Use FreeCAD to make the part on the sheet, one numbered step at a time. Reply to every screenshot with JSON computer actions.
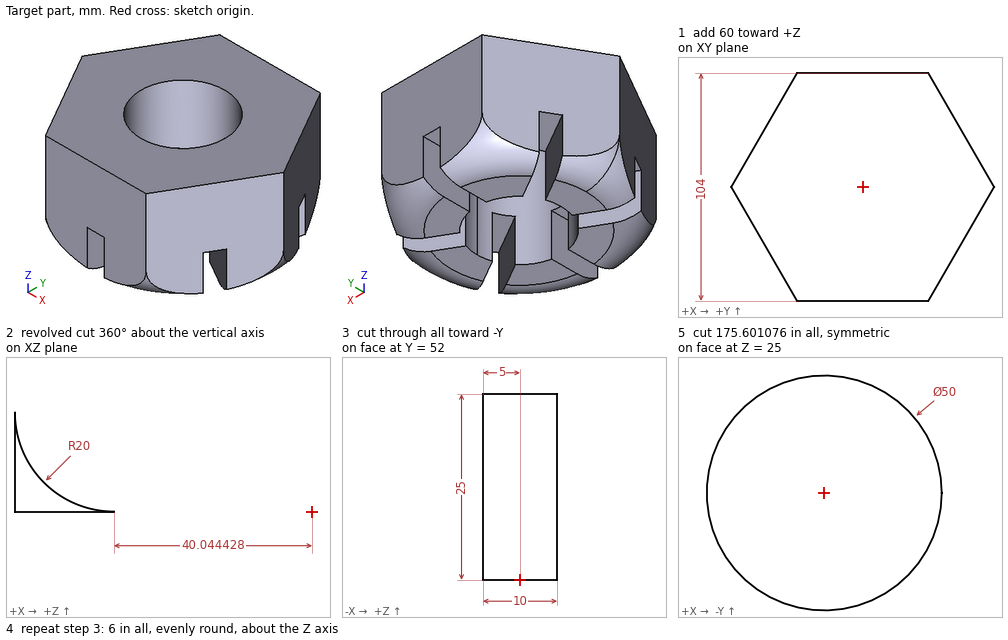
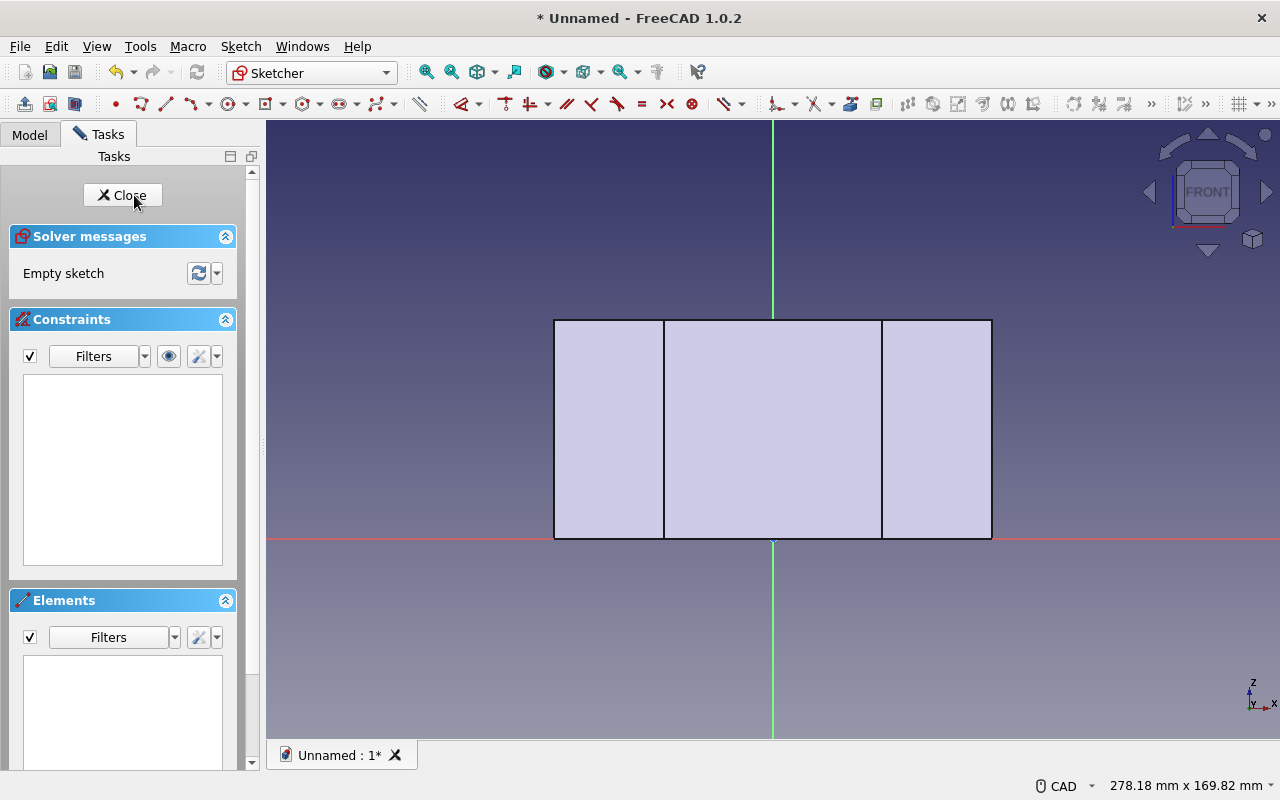
{"action": "left_click", "coordinate": [75, 104]}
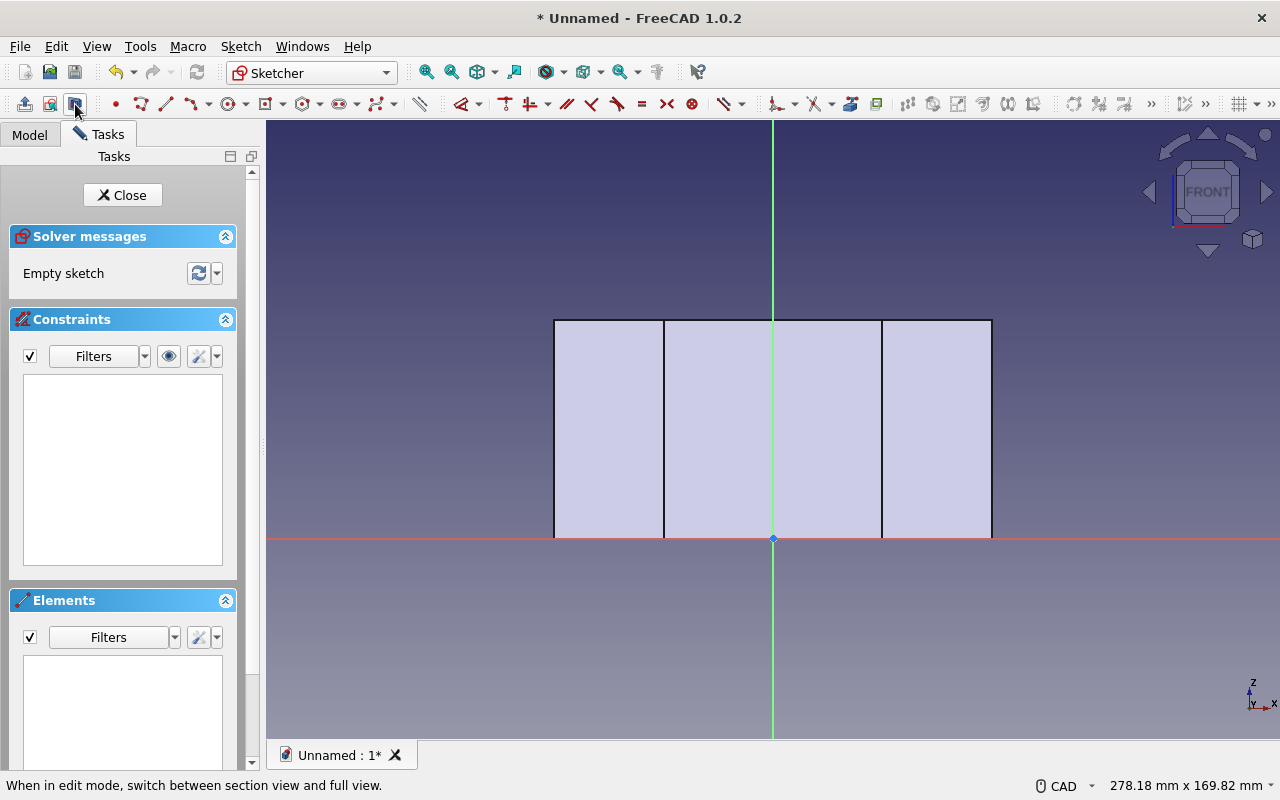
{"action": "scroll", "coordinate": [562, 521], "scroll_direction": "up", "scroll_amount": 8}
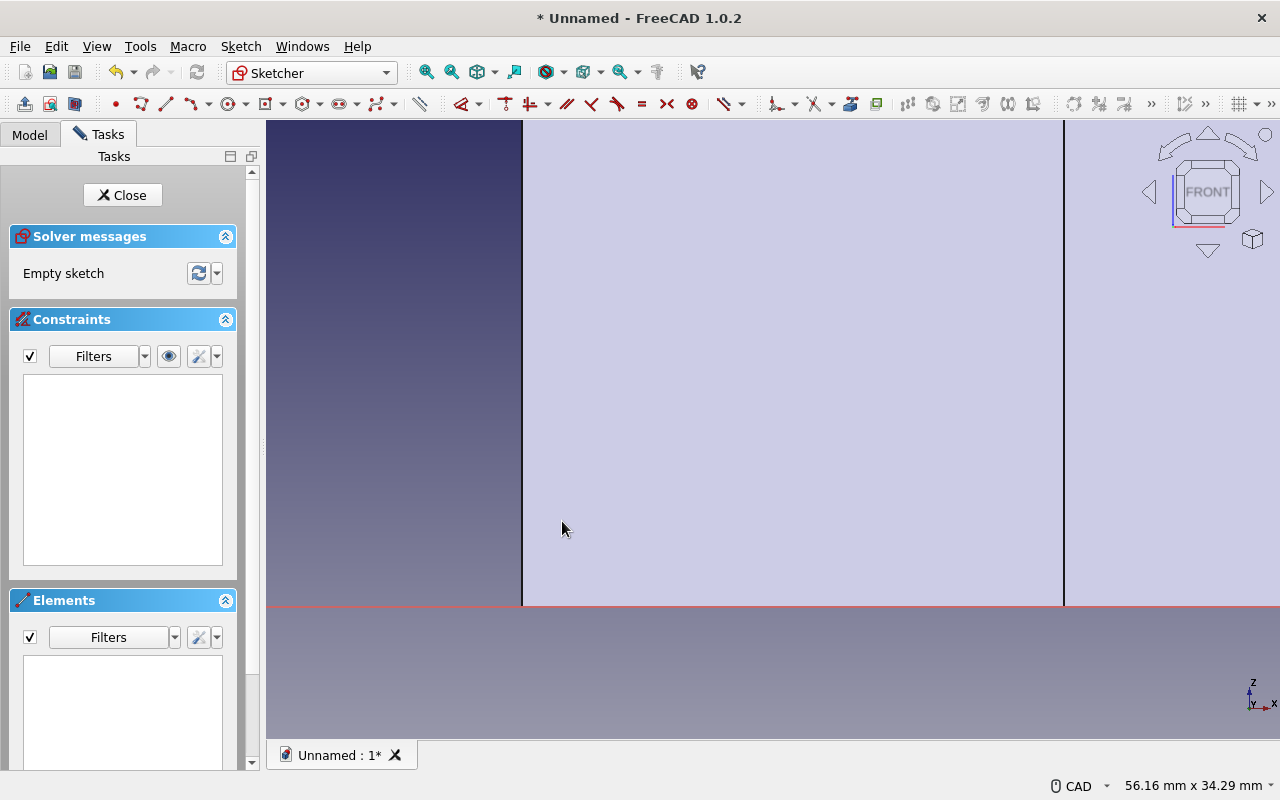
{"action": "left_click", "coordinate": [141, 104]}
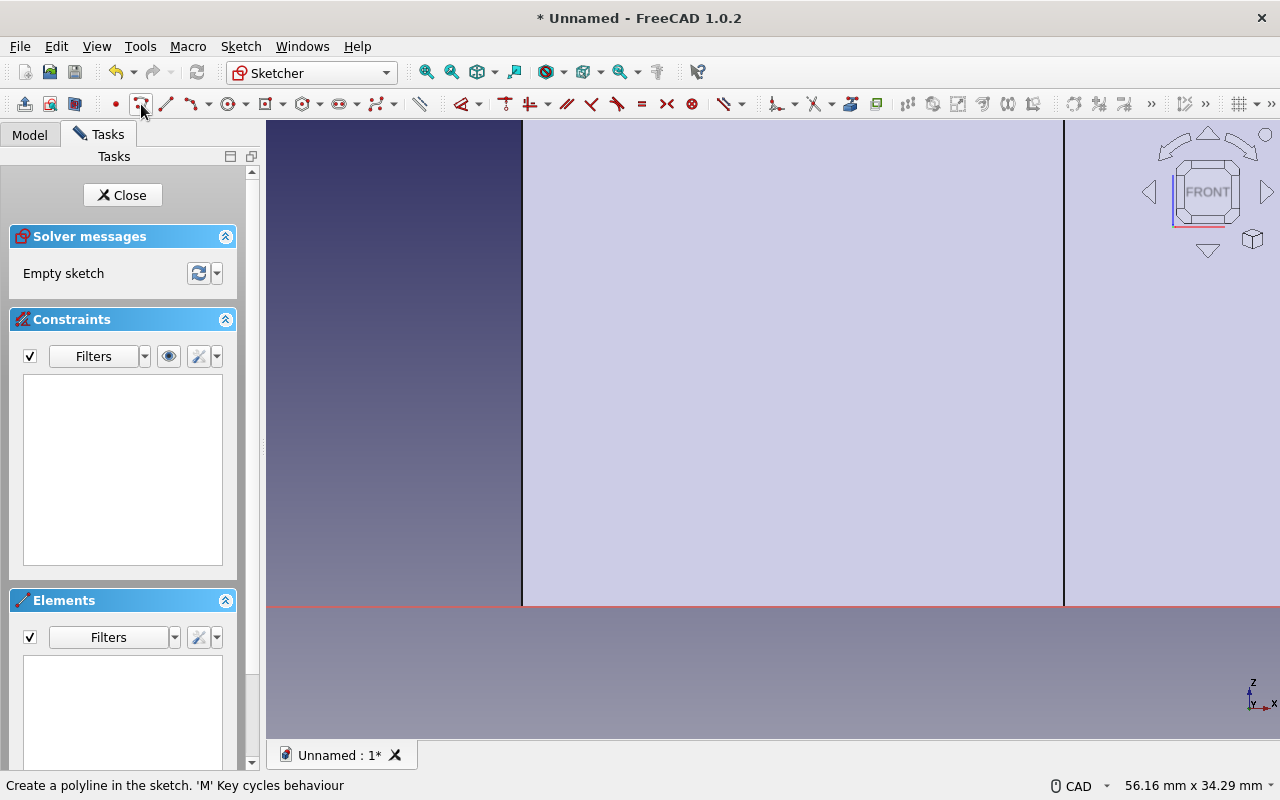
{"action": "left_click", "coordinate": [883, 607]}
{"action": "left_click", "coordinate": [522, 598]}
{"action": "left_click", "coordinate": [522, 246]}
{"action": "right_click", "coordinate": [522, 246]}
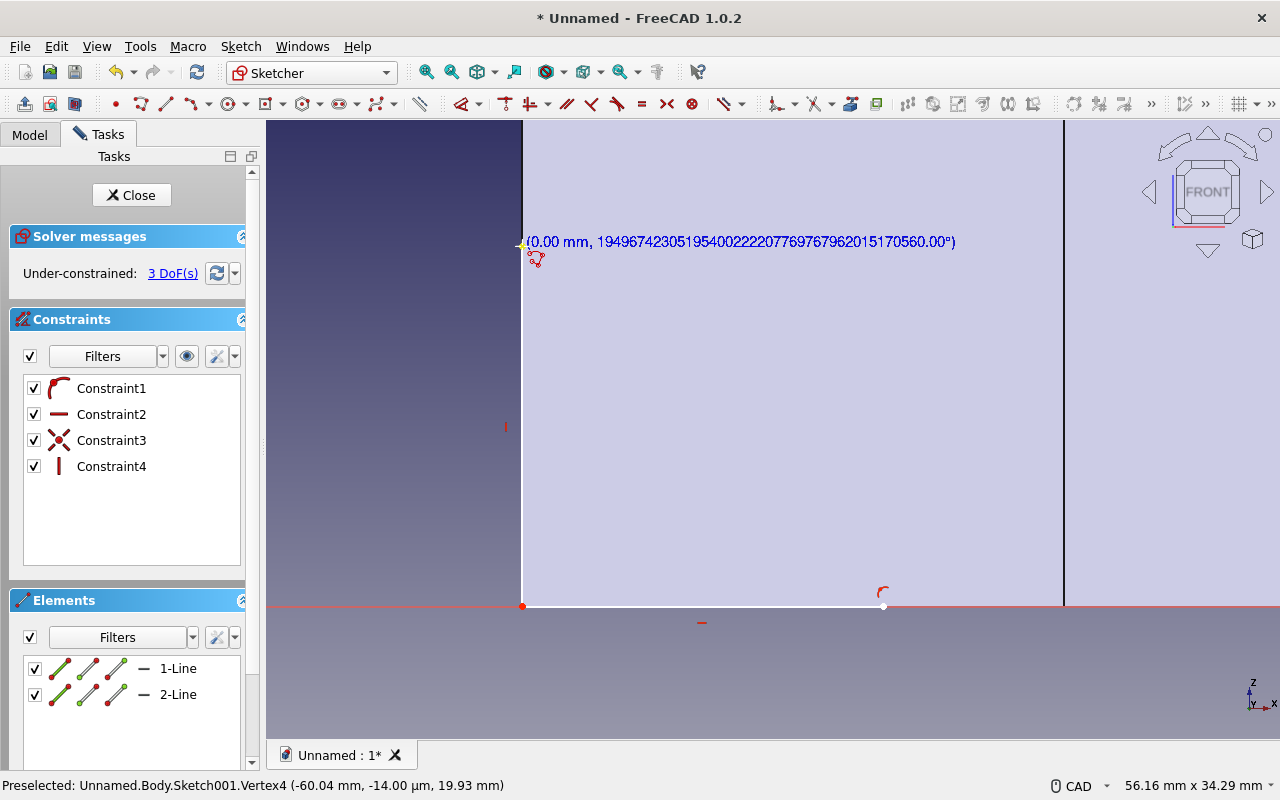
{"action": "key", "text": "g 3 a"}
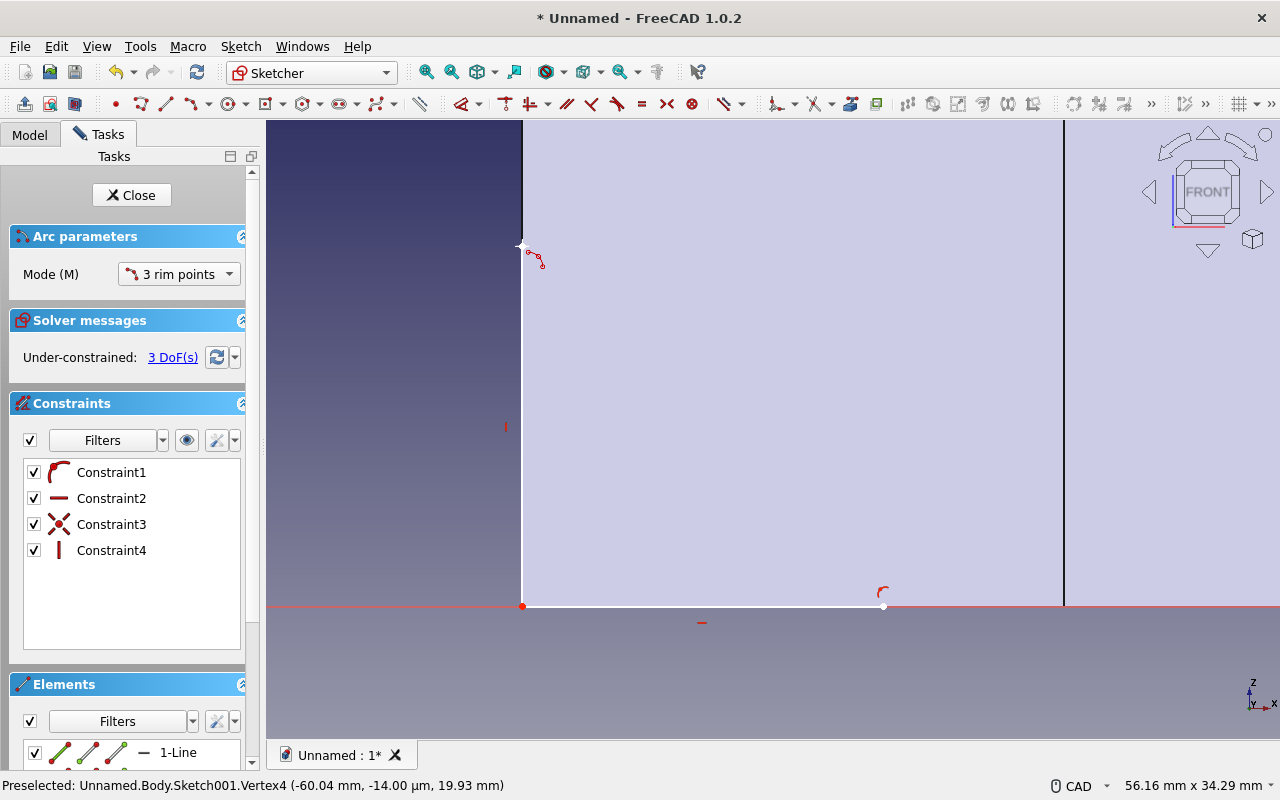
{"action": "left_click", "coordinate": [522, 247]}
{"action": "left_click", "coordinate": [883, 607]}
{"action": "left_click", "coordinate": [628, 501]}
{"action": "key", "text": "Escape"}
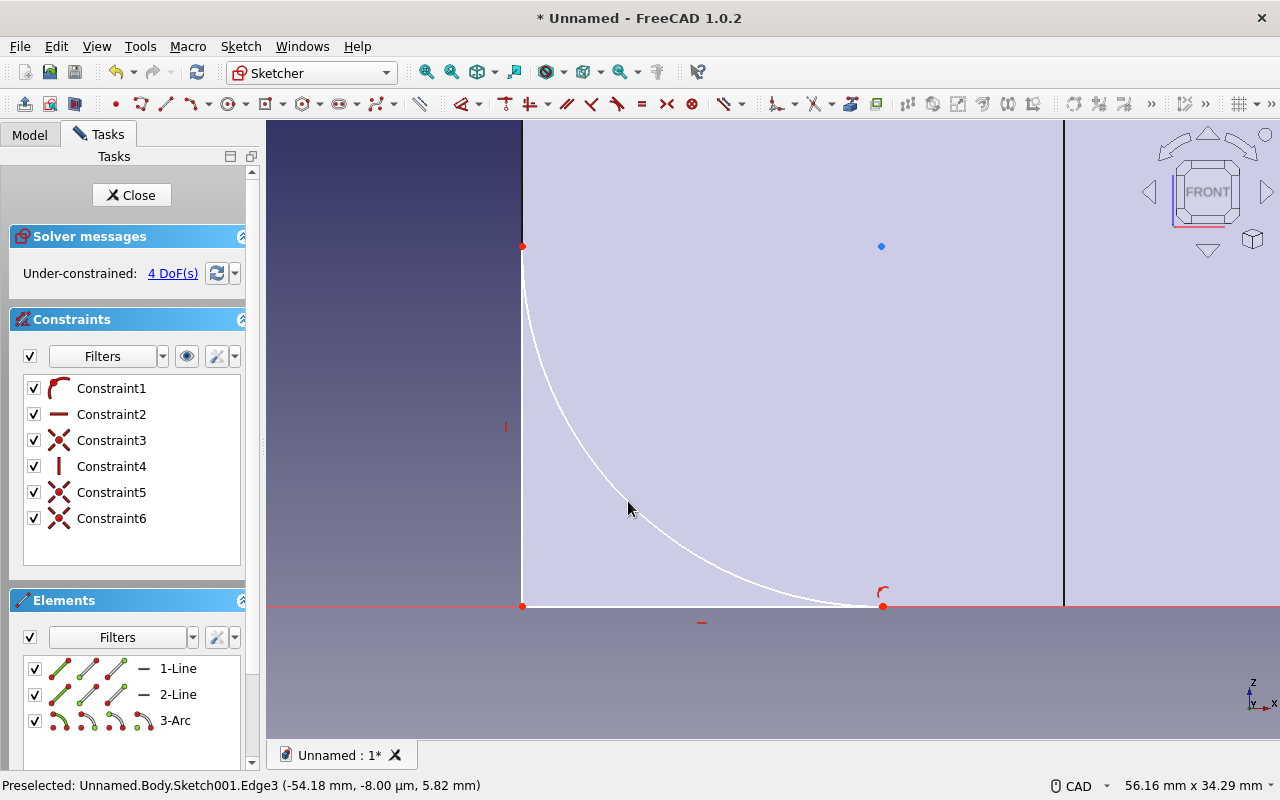
{"action": "left_click", "coordinate": [775, 607]}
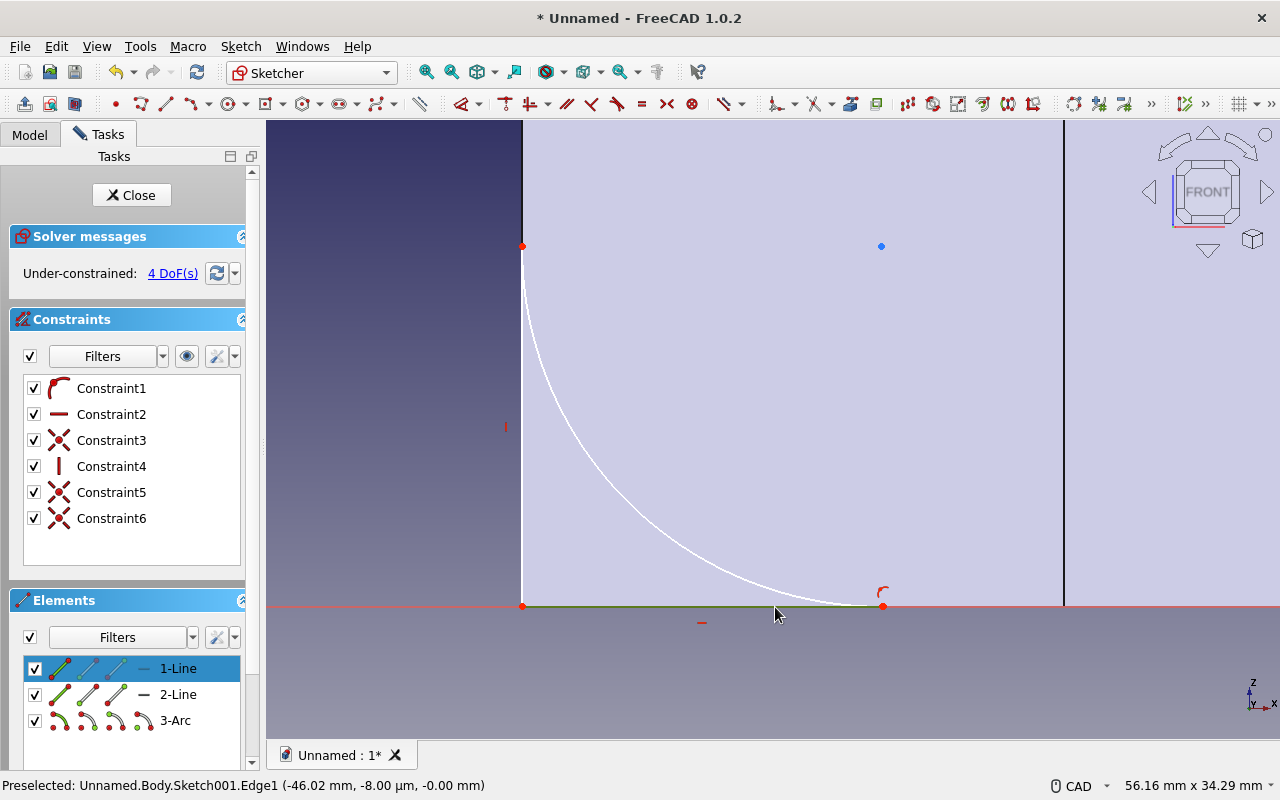
{"action": "left_click", "coordinate": [561, 411]}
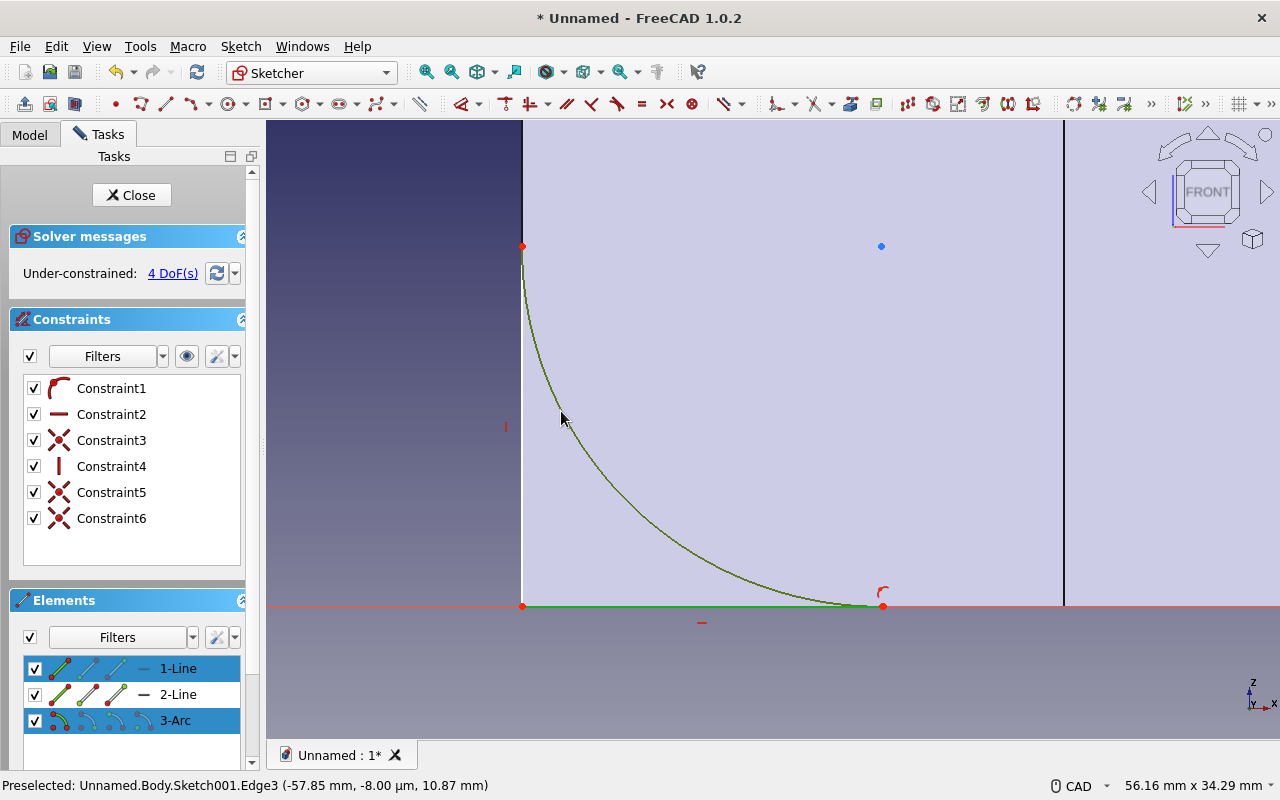
{"action": "key", "text": "t"}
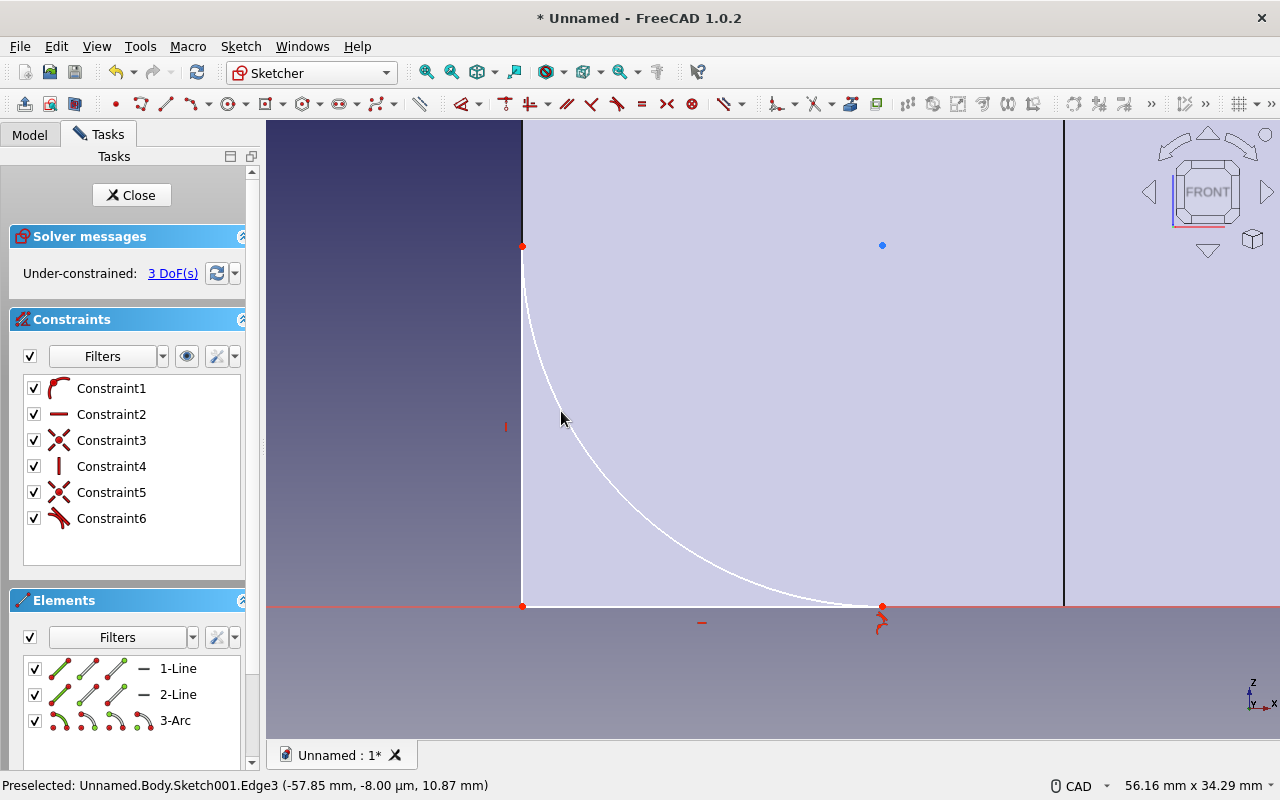
{"action": "left_click", "coordinate": [522, 499]}